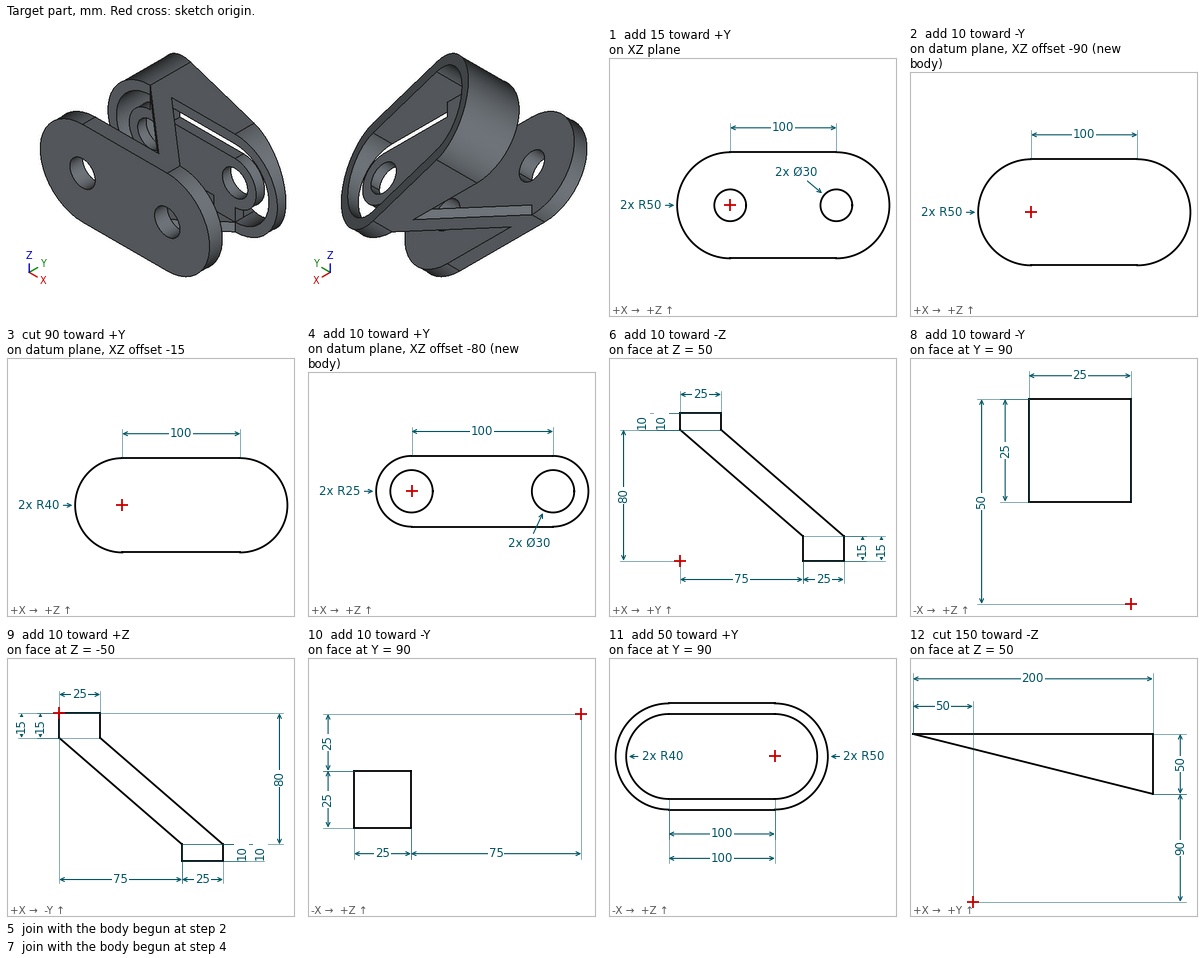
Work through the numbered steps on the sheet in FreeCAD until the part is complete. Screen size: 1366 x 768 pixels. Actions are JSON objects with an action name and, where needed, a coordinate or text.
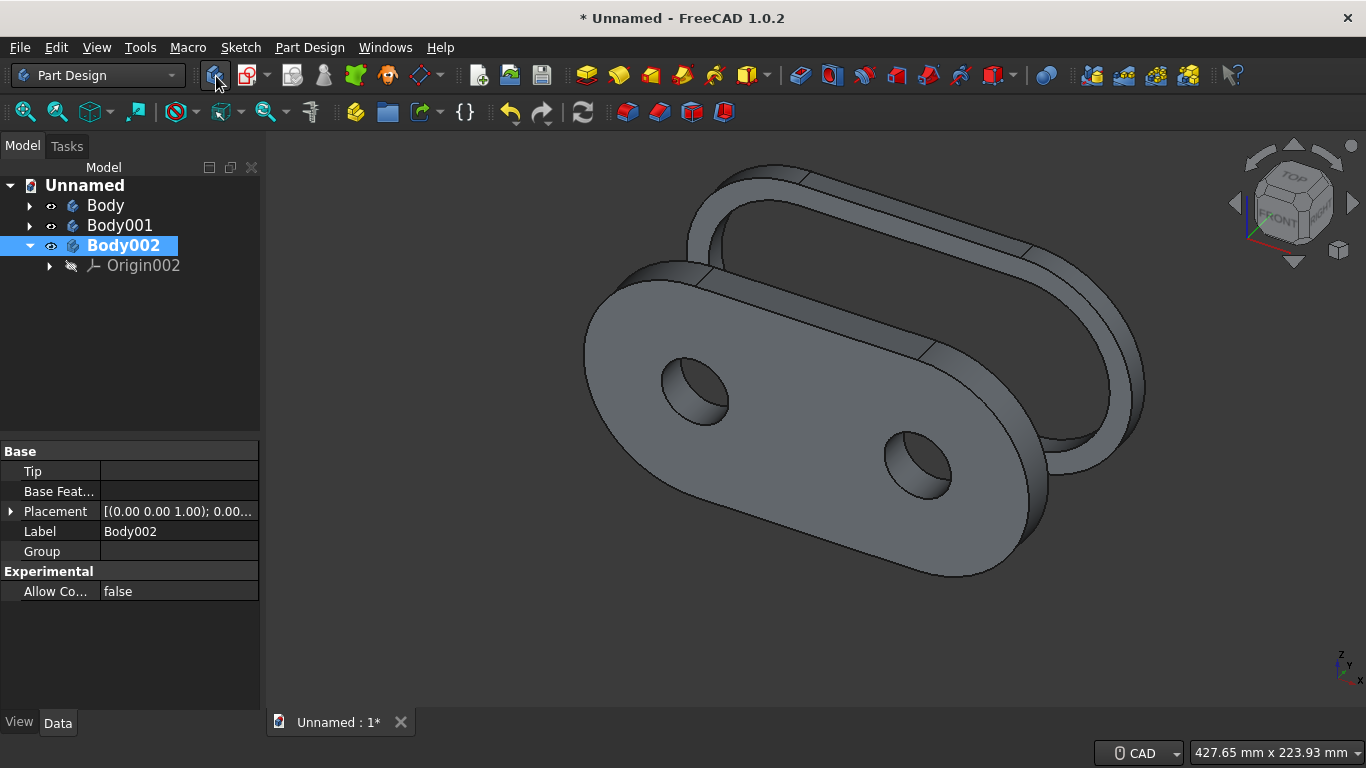
{"action": "left_click", "coordinate": [50, 266]}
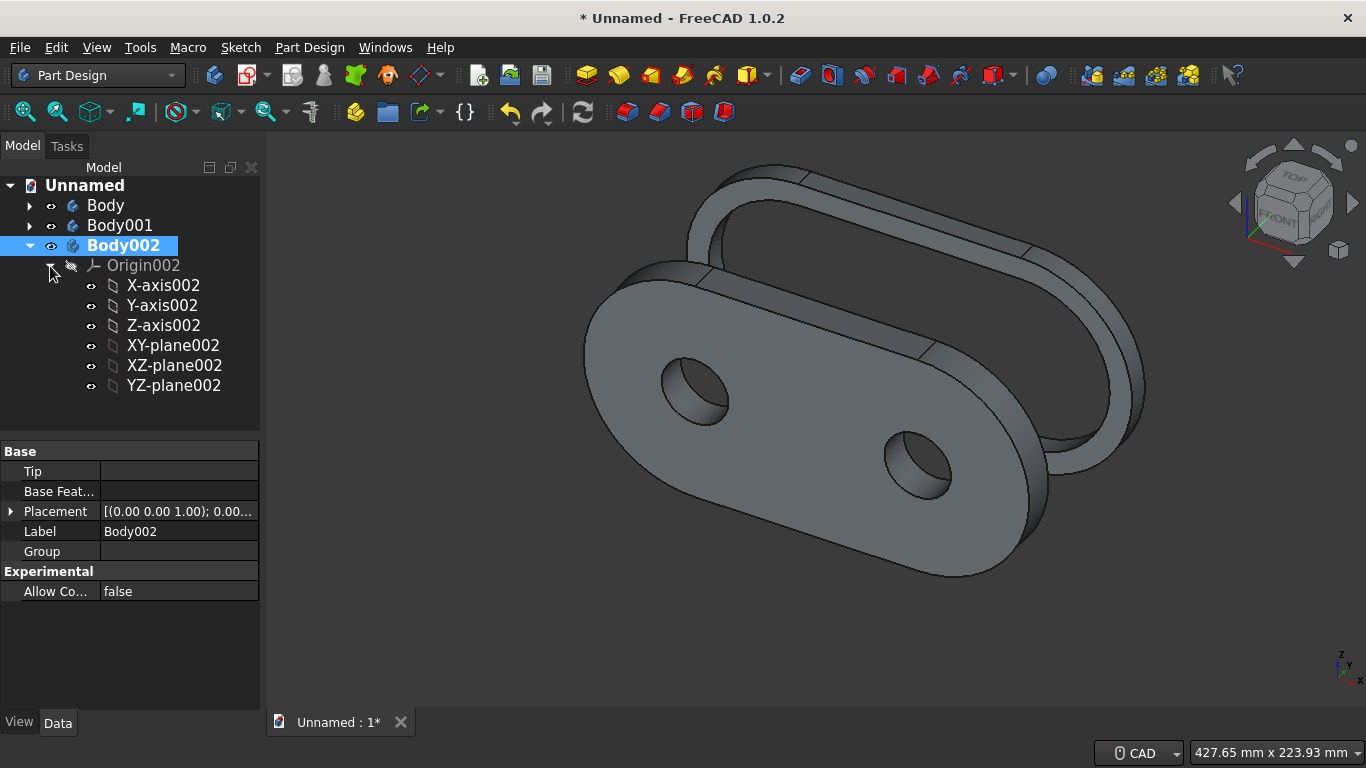
{"action": "left_click", "coordinate": [136, 366]}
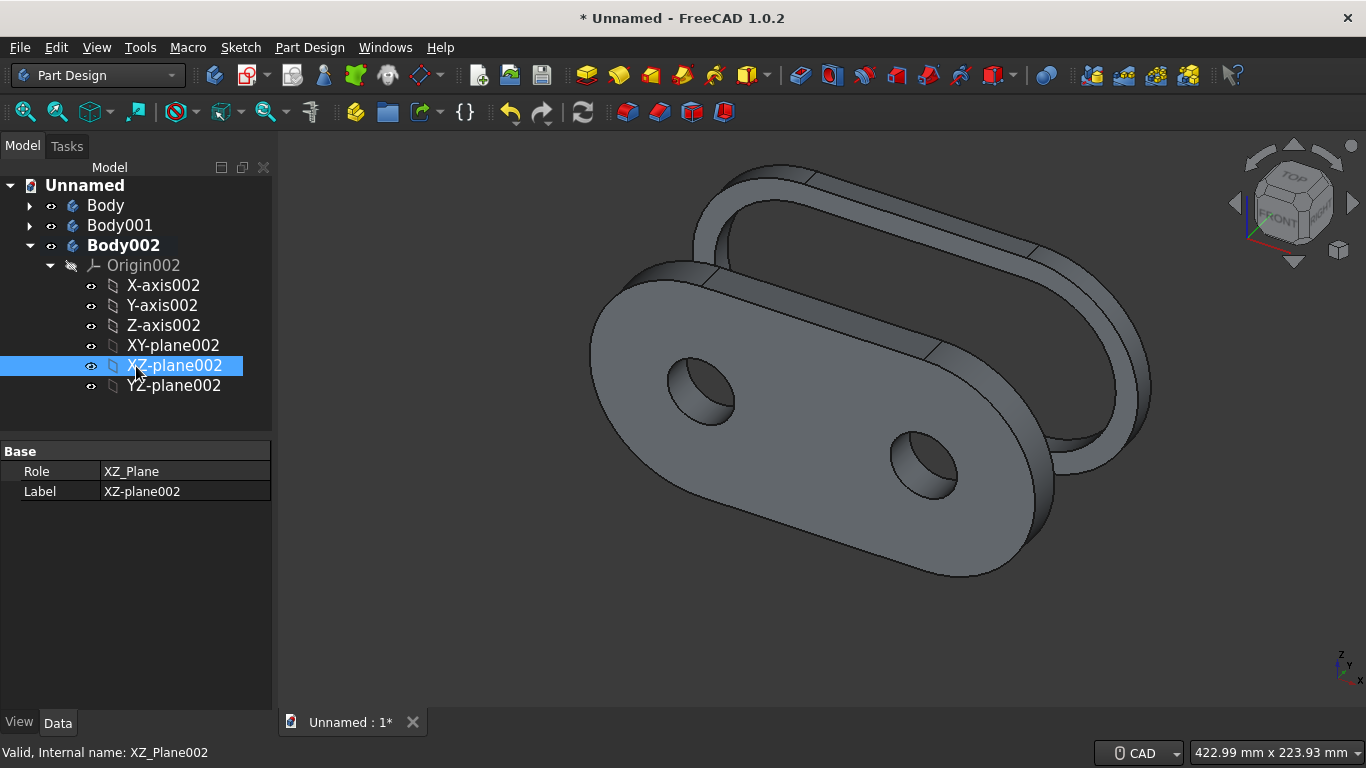
{"action": "left_click", "coordinate": [420, 76]}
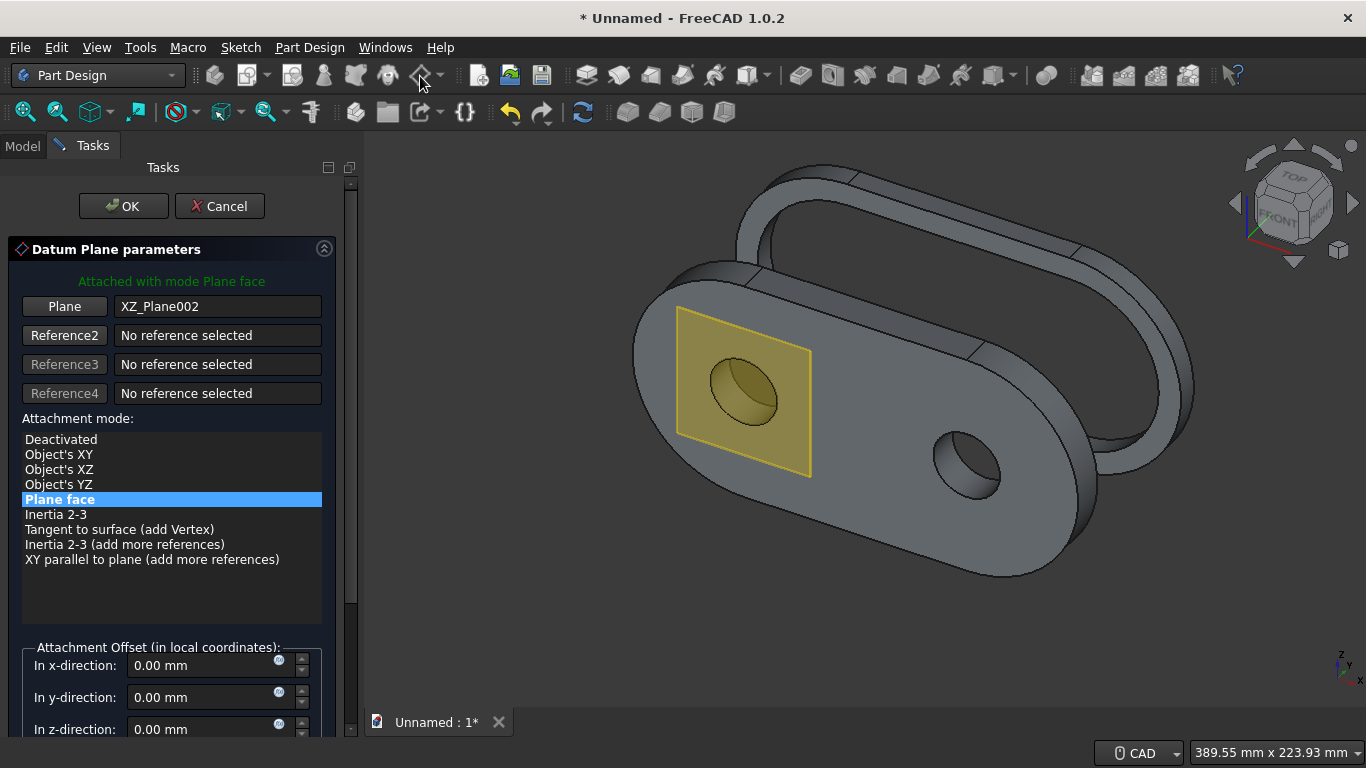
{"action": "scroll", "coordinate": [351, 456], "scroll_direction": "down", "scroll_amount": 2}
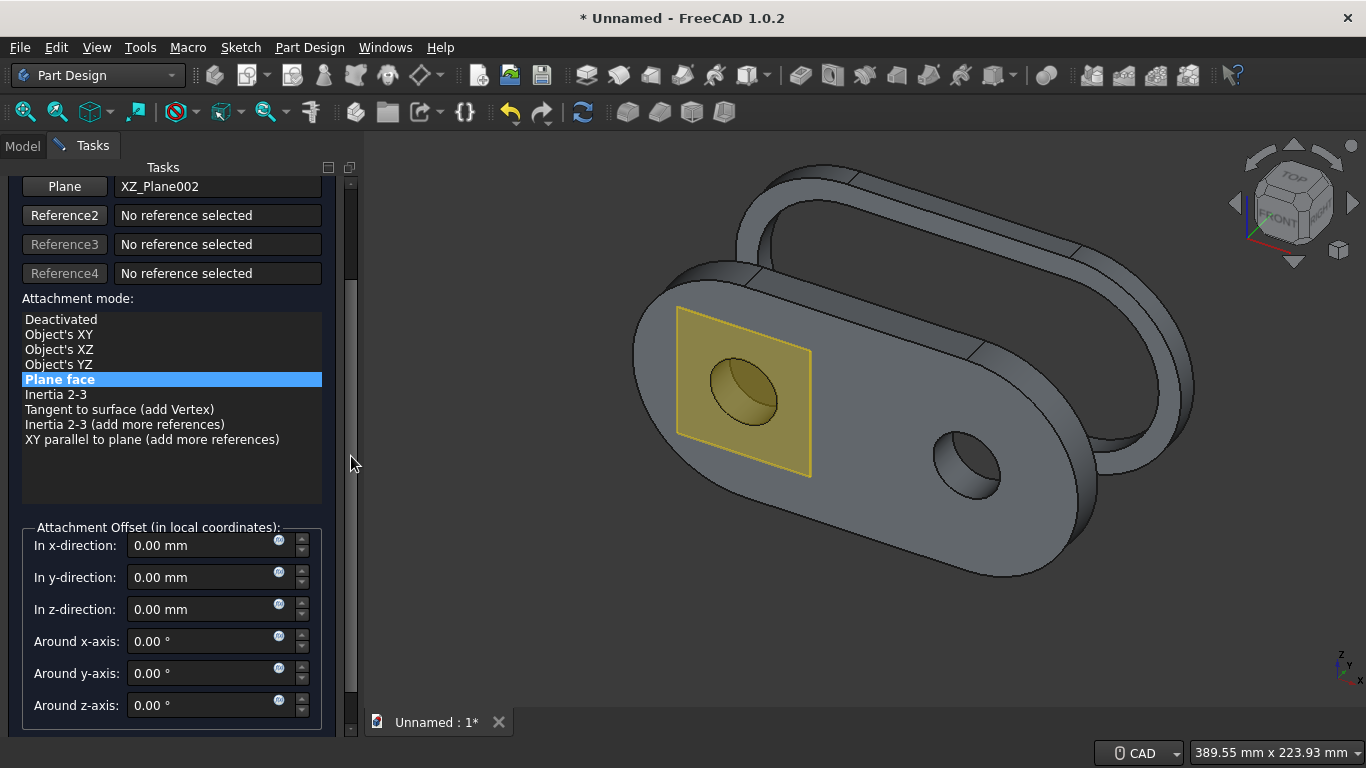
{"action": "triple_click", "coordinate": [210, 609]}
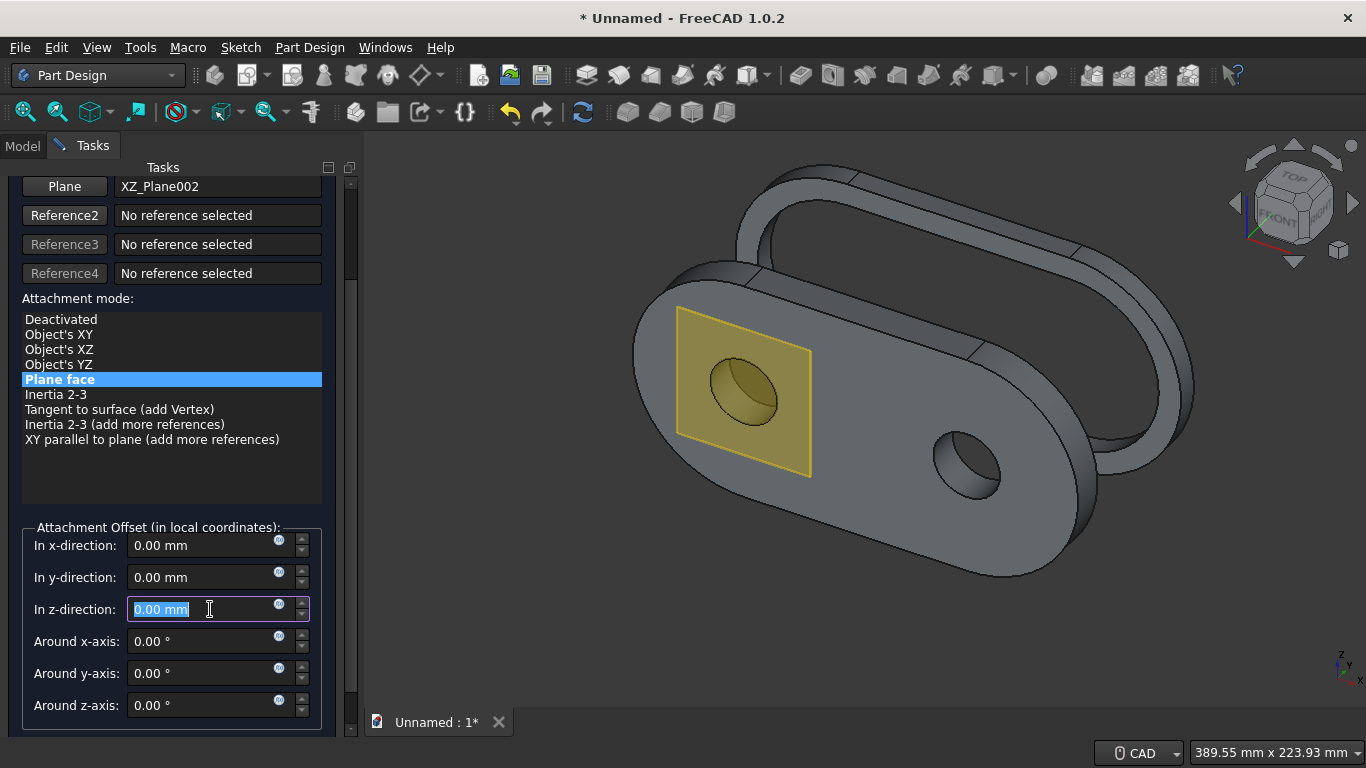
{"action": "type", "text": "-80"}
{"action": "key", "text": "Tab"}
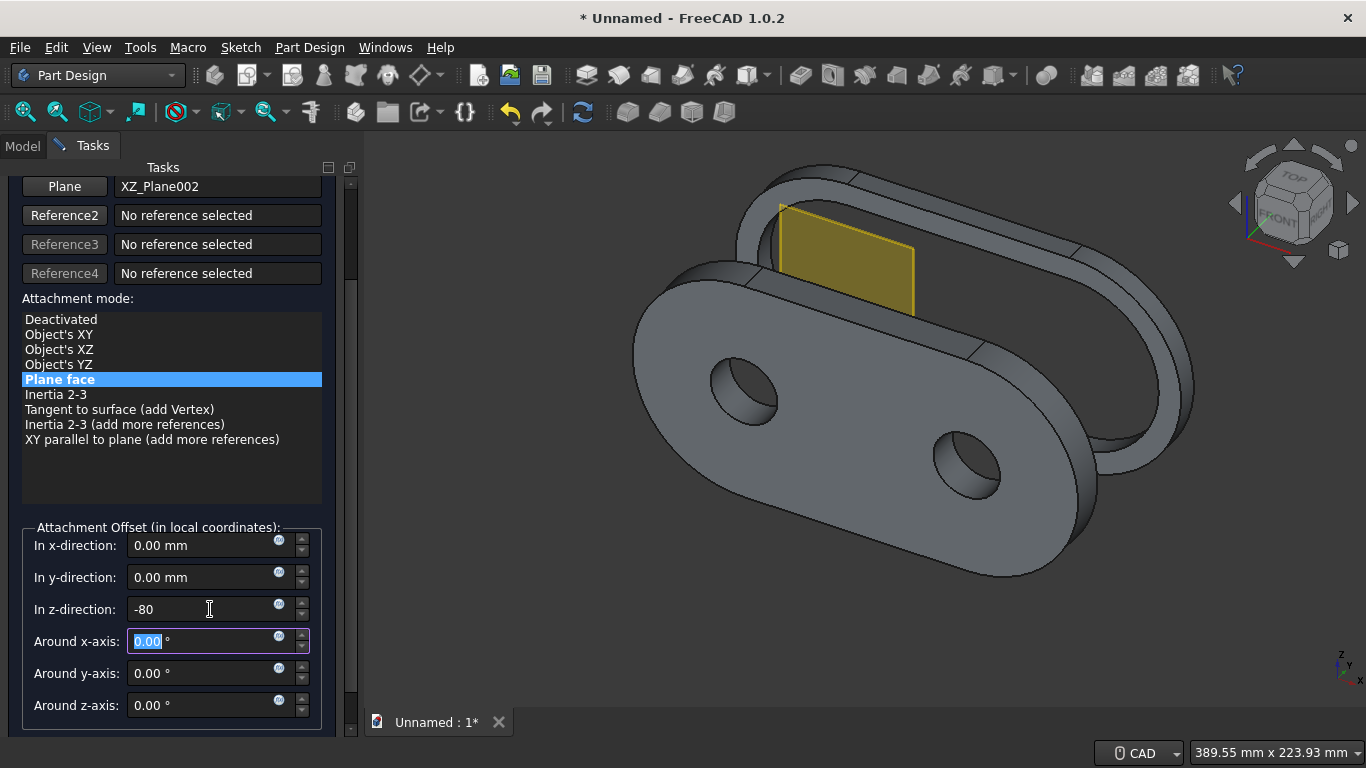
{"action": "scroll", "coordinate": [351, 456], "scroll_direction": "up", "scroll_amount": 3}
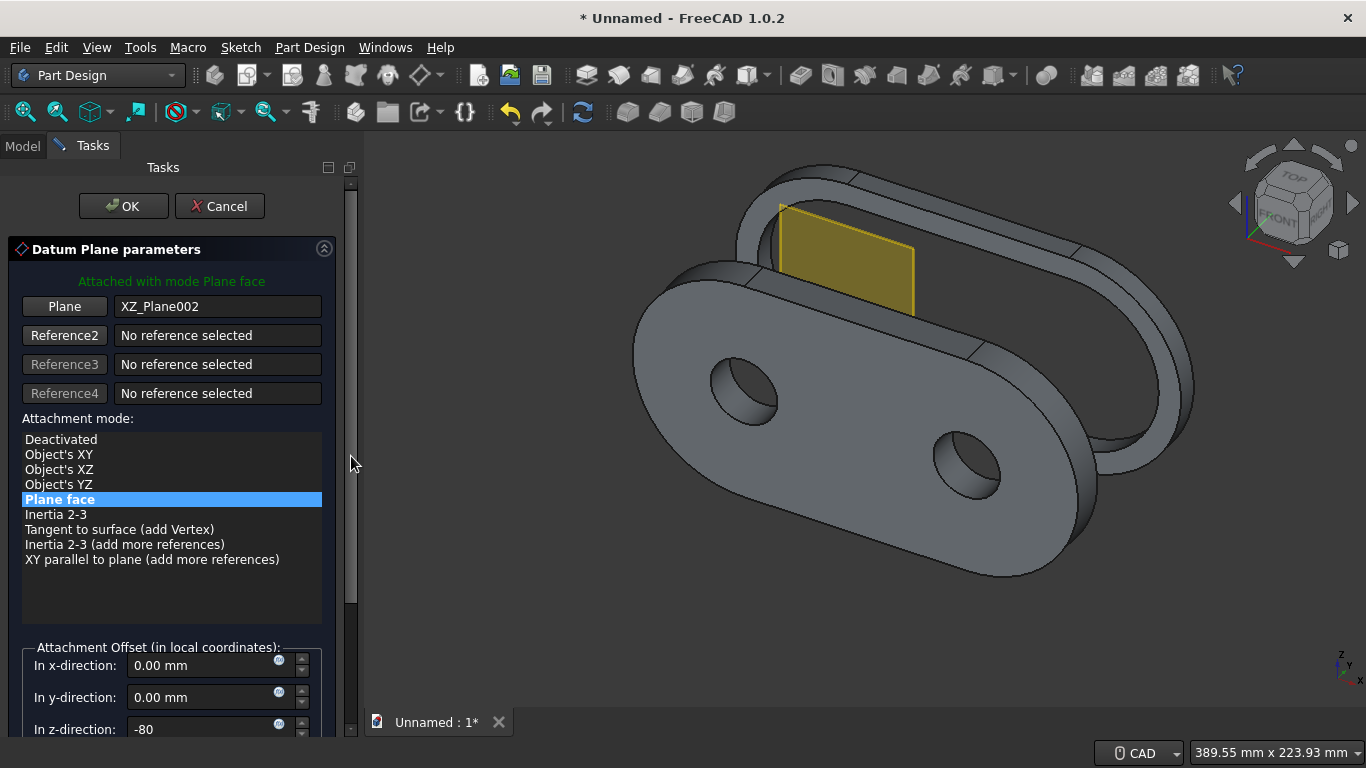
{"action": "left_click", "coordinate": [124, 206]}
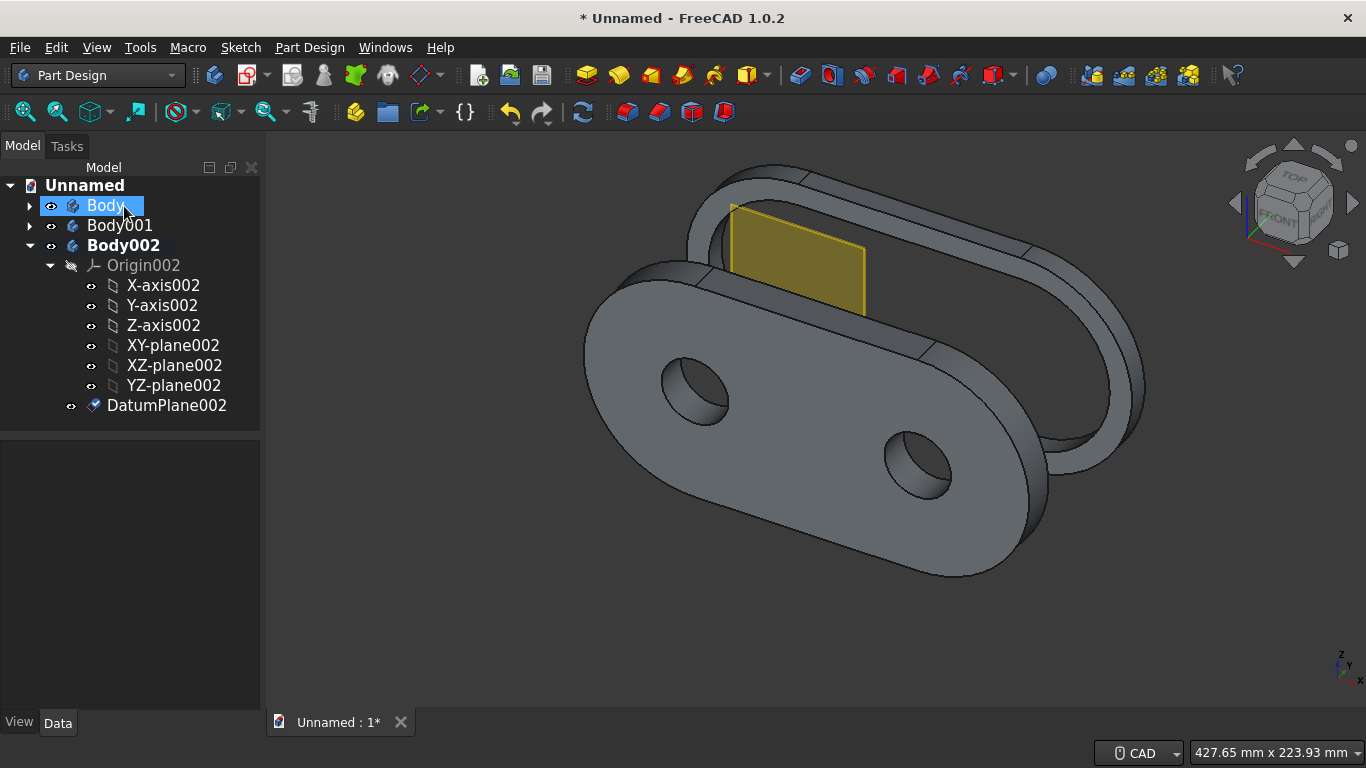
{"action": "left_click", "coordinate": [116, 406]}